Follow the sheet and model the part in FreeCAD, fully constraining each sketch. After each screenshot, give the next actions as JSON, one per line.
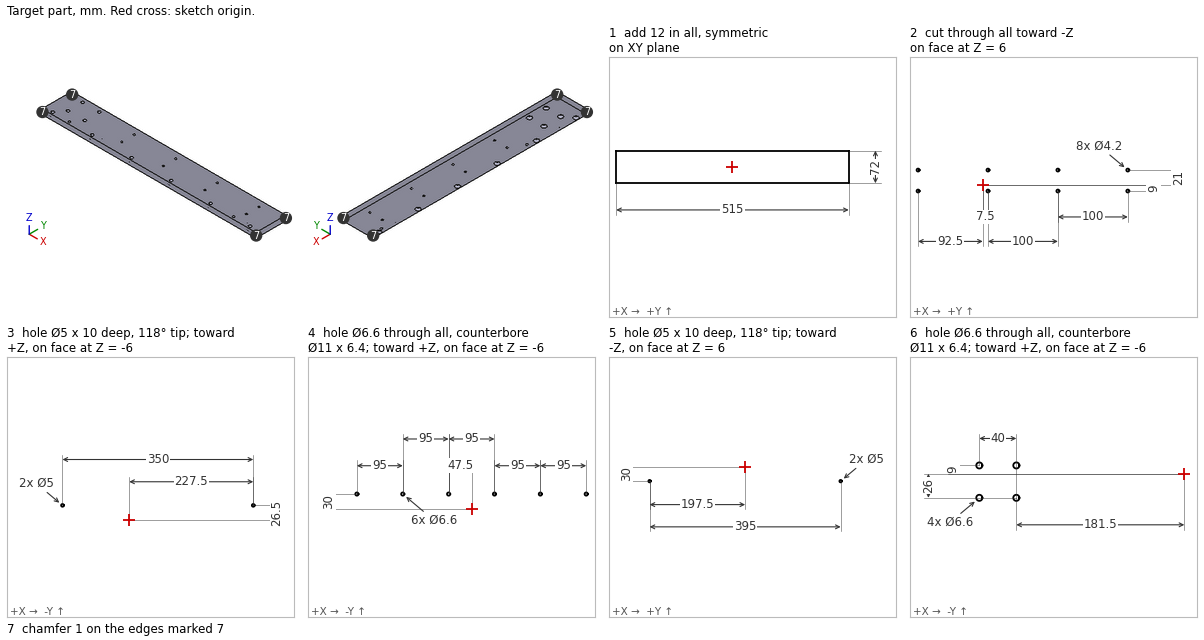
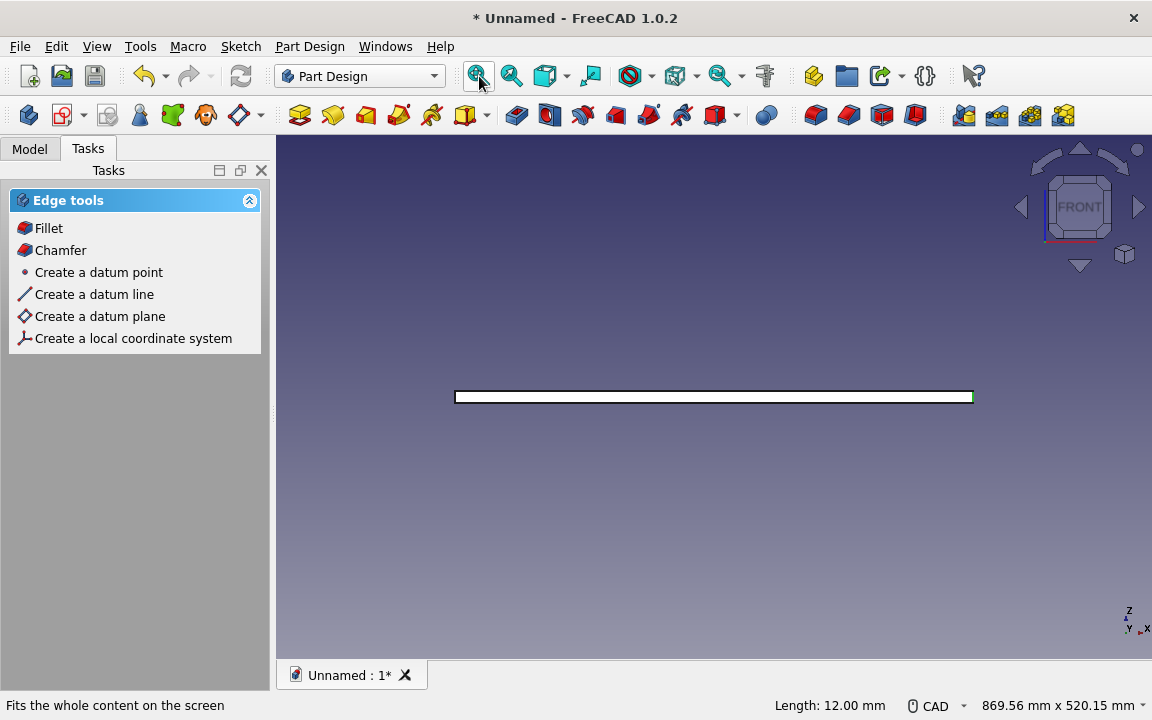
{"action": "left_click", "coordinate": [455, 396], "text": "ctrl"}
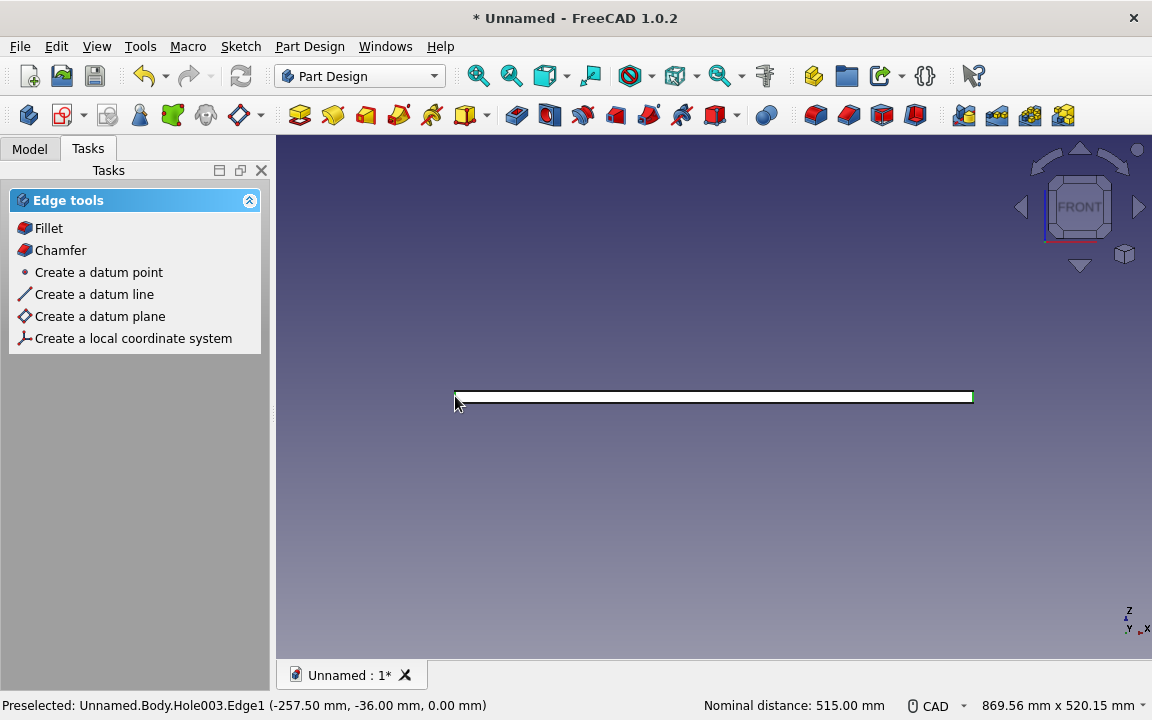
{"action": "scroll", "coordinate": [455, 396], "scroll_direction": "up", "scroll_amount": 6}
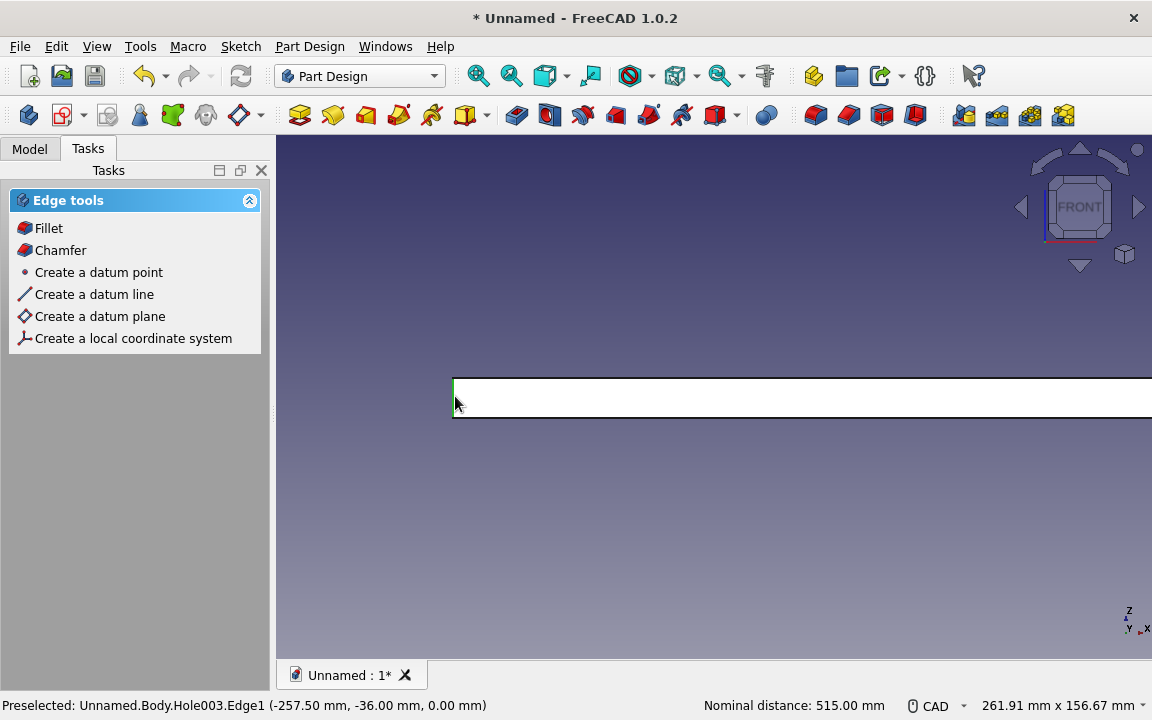
{"action": "left_click", "coordinate": [479, 76]}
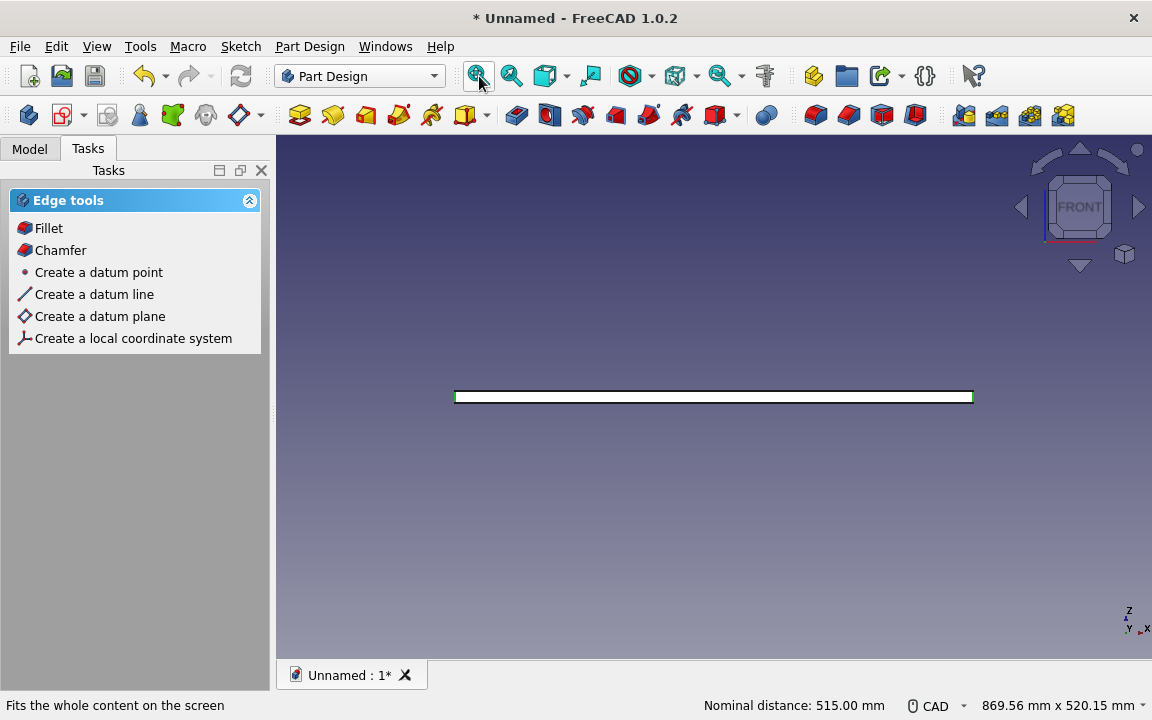
{"action": "key", "text": "3"}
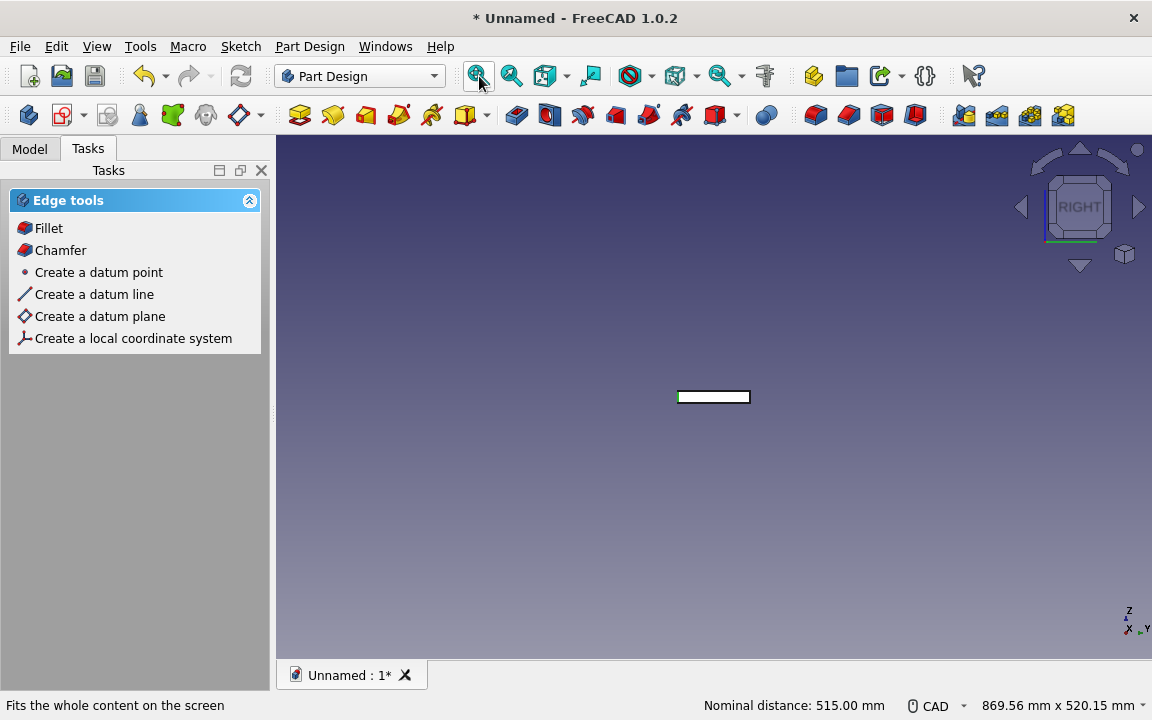
{"action": "left_click", "coordinate": [479, 76]}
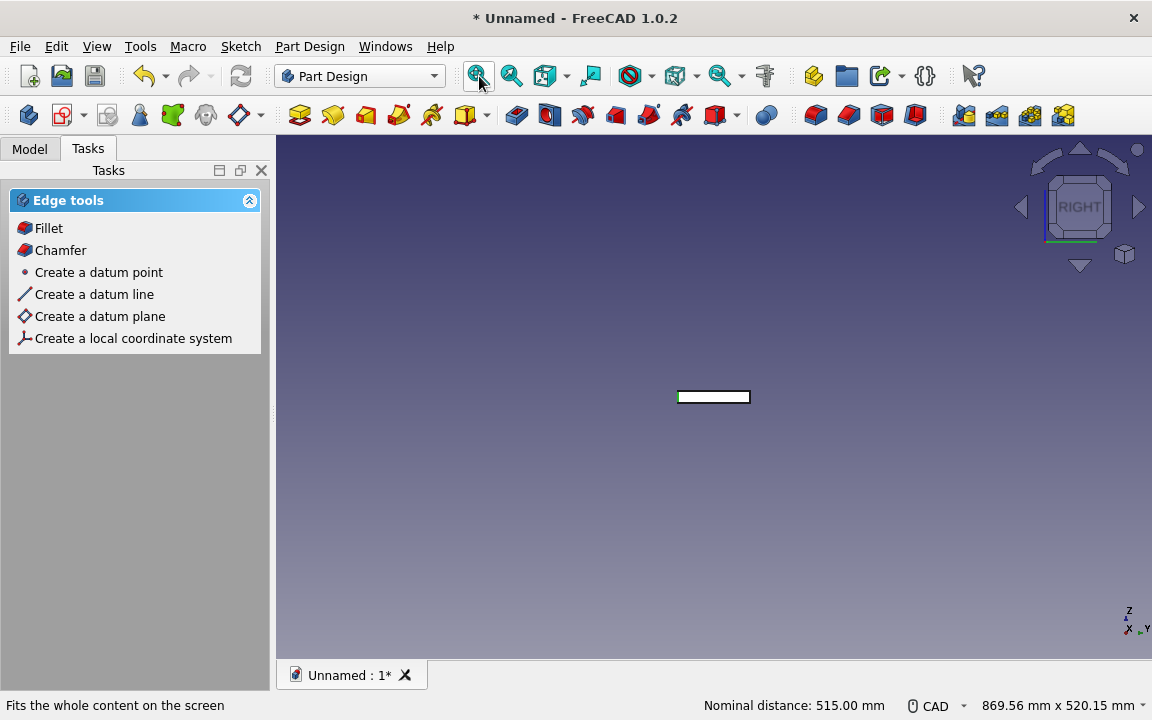
{"action": "left_click", "coordinate": [750, 396], "text": "ctrl"}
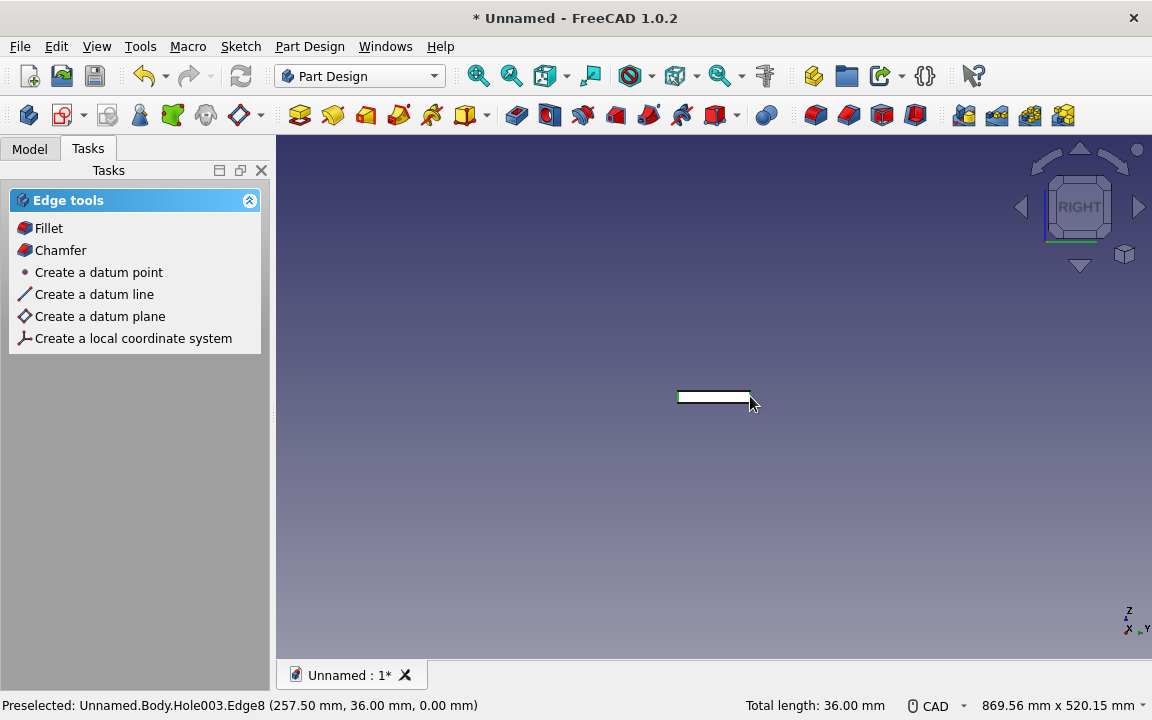
{"action": "scroll", "coordinate": [750, 396], "scroll_direction": "up", "scroll_amount": 6}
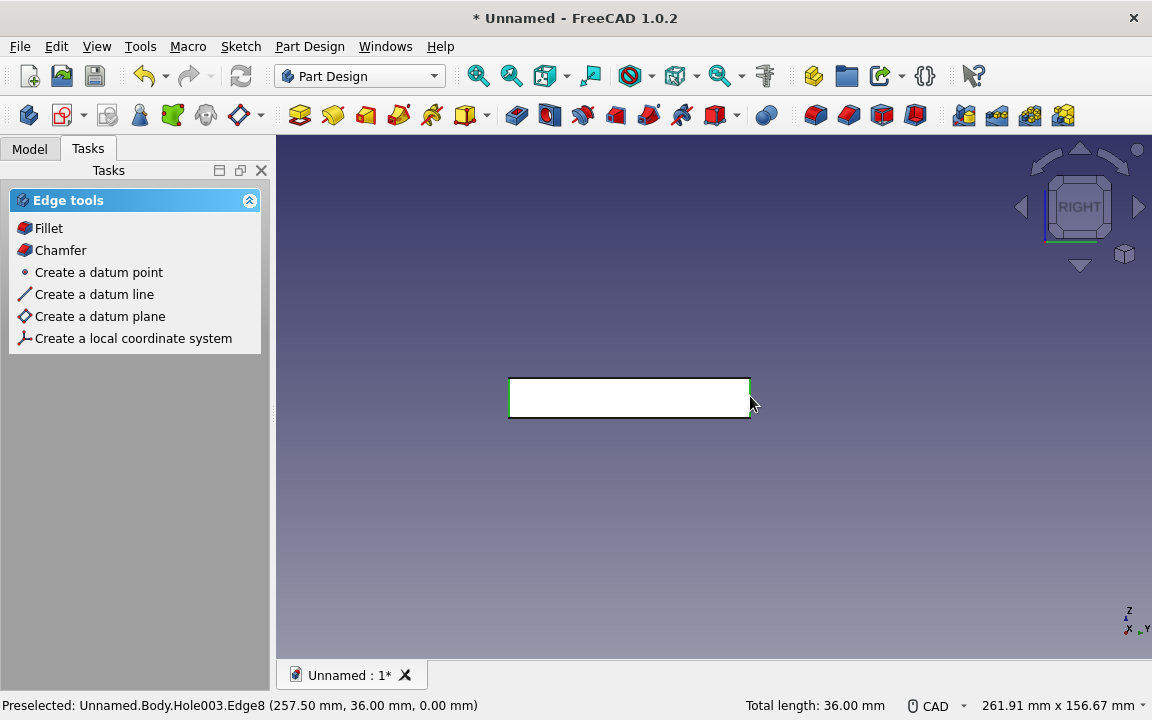
{"action": "left_click", "coordinate": [479, 76]}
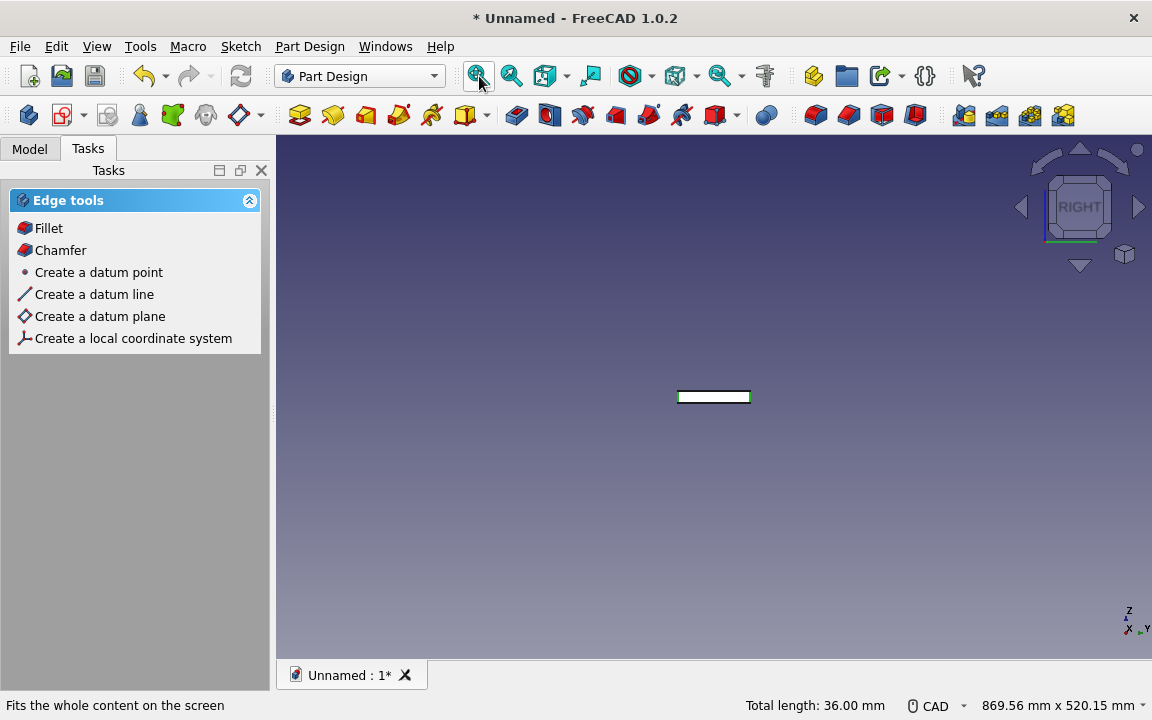
{"action": "key", "text": "5"}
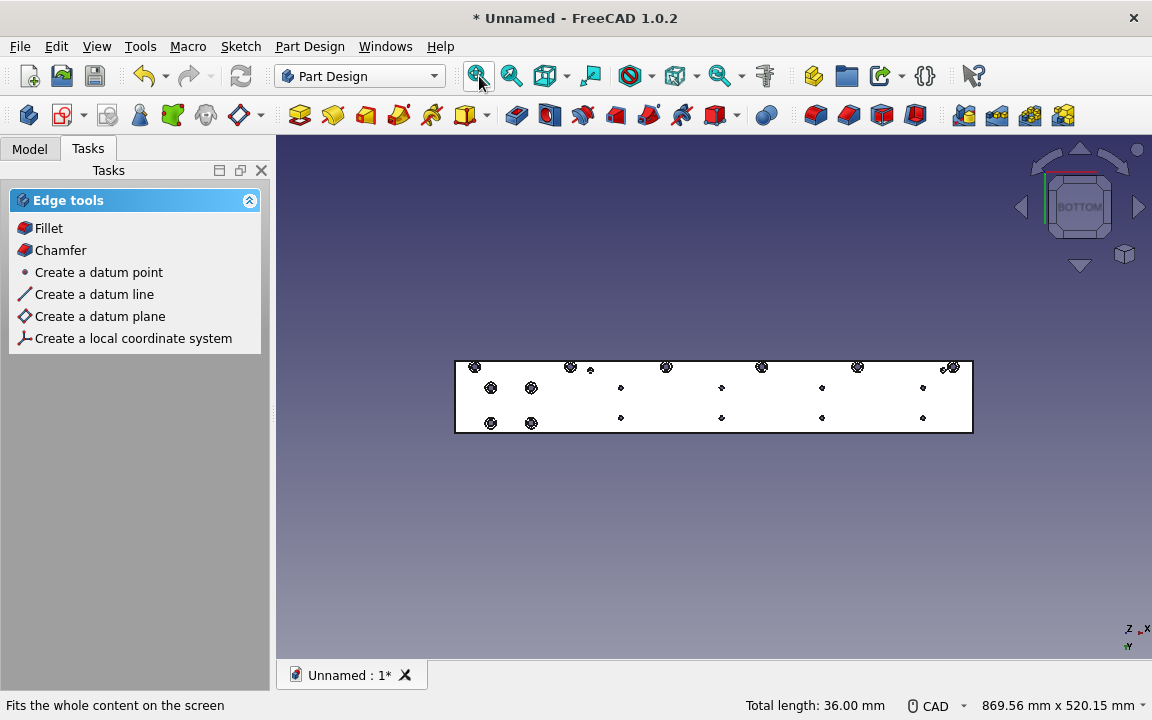
{"action": "scroll", "coordinate": [455, 432], "scroll_direction": "up", "scroll_amount": 6}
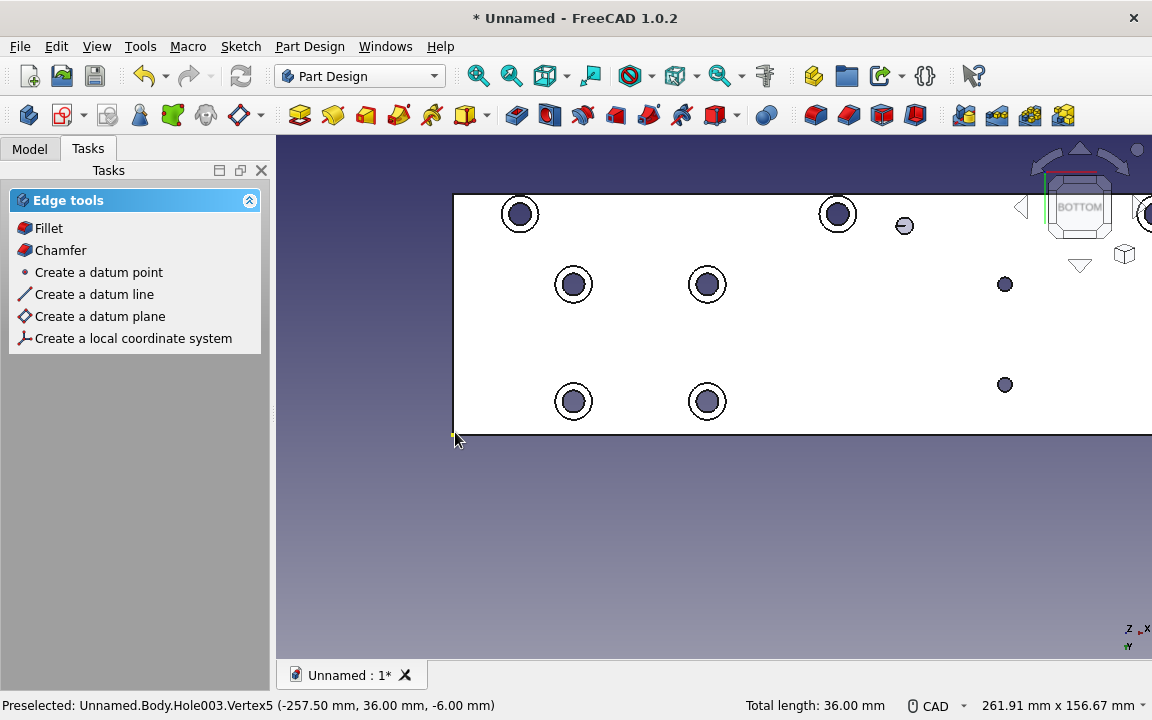
{"action": "left_click", "coordinate": [479, 76]}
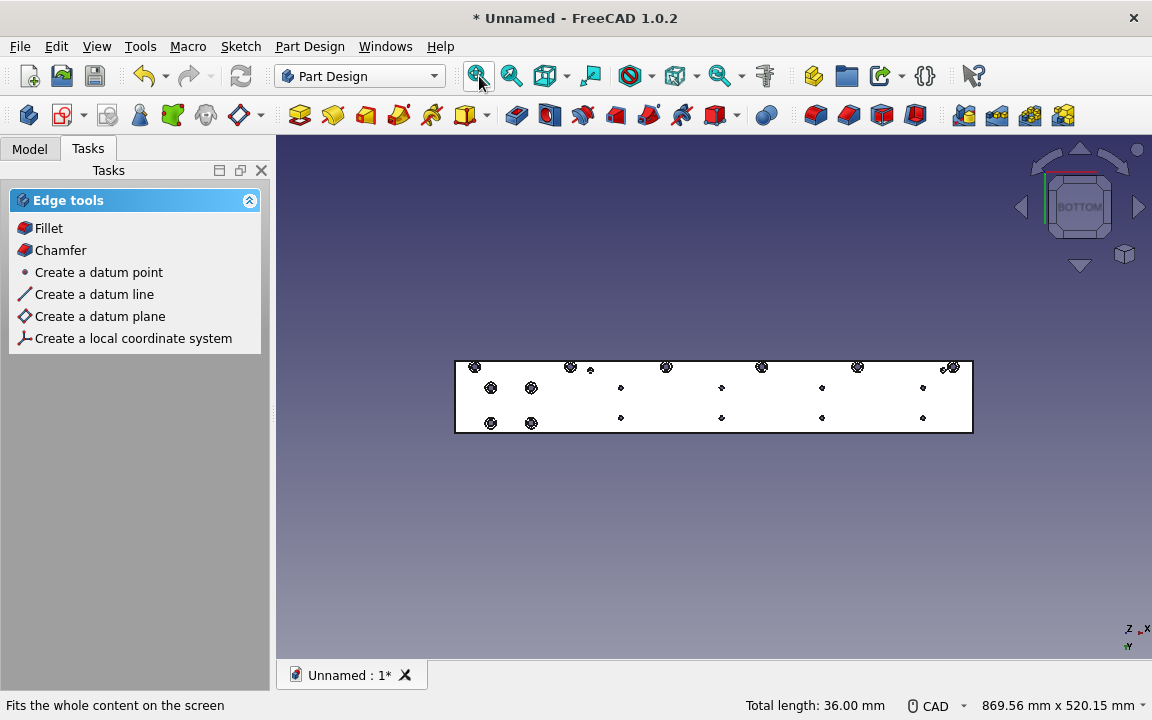
{"action": "key", "text": "4"}